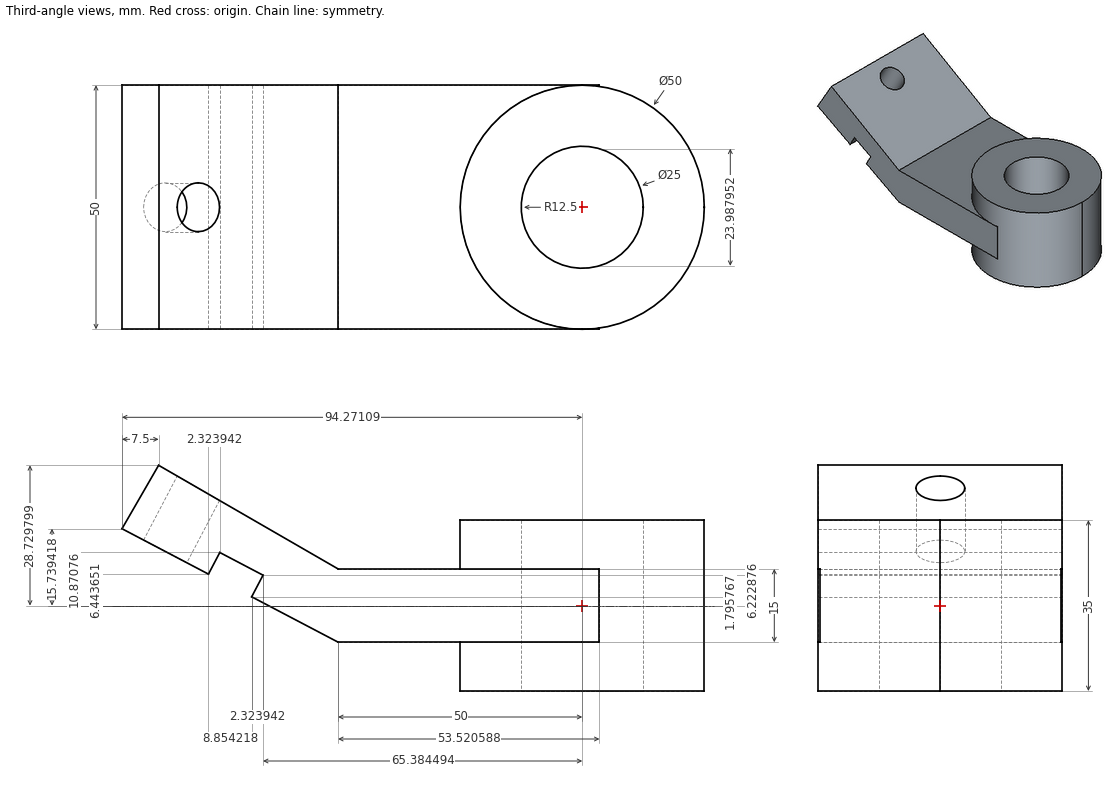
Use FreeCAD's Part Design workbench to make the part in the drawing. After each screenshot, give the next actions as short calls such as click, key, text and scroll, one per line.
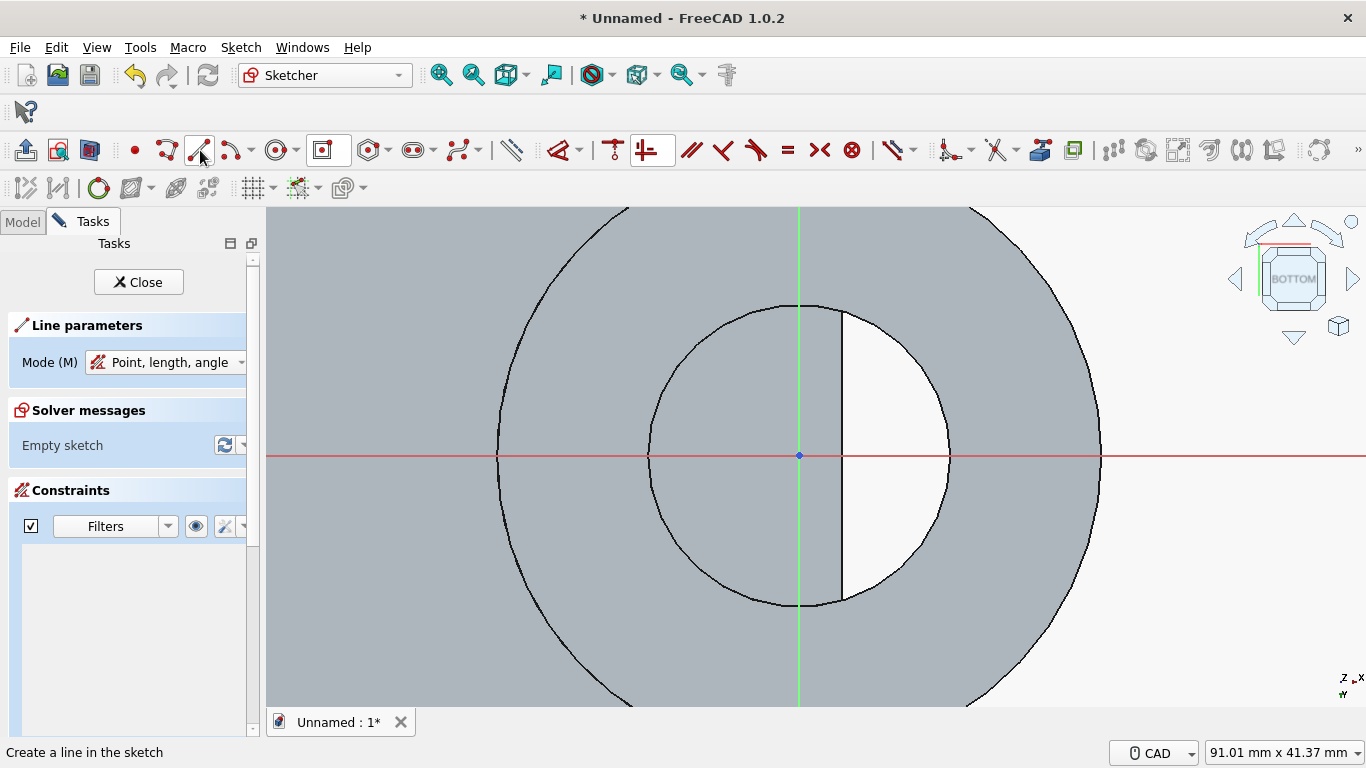
click(842, 601)
click(842, 311)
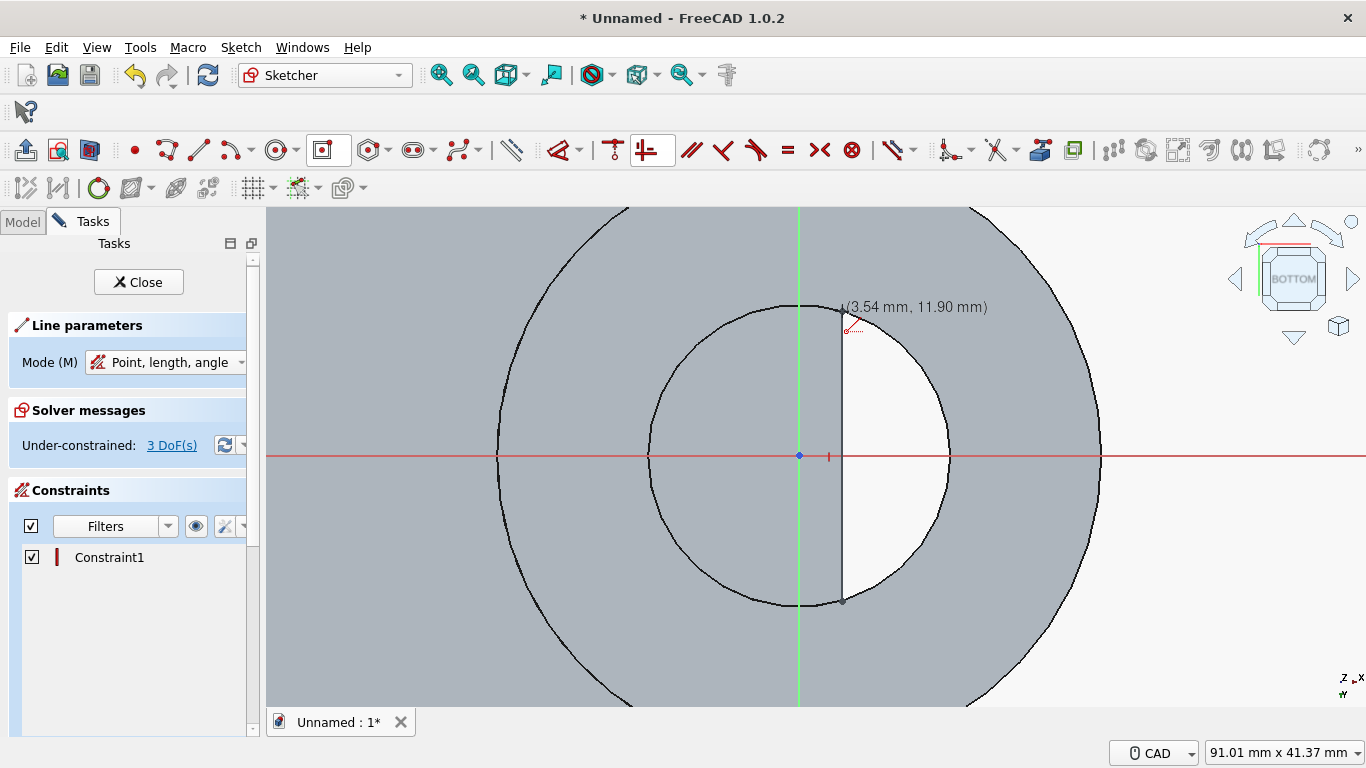
key(g)
key(3)
key(a)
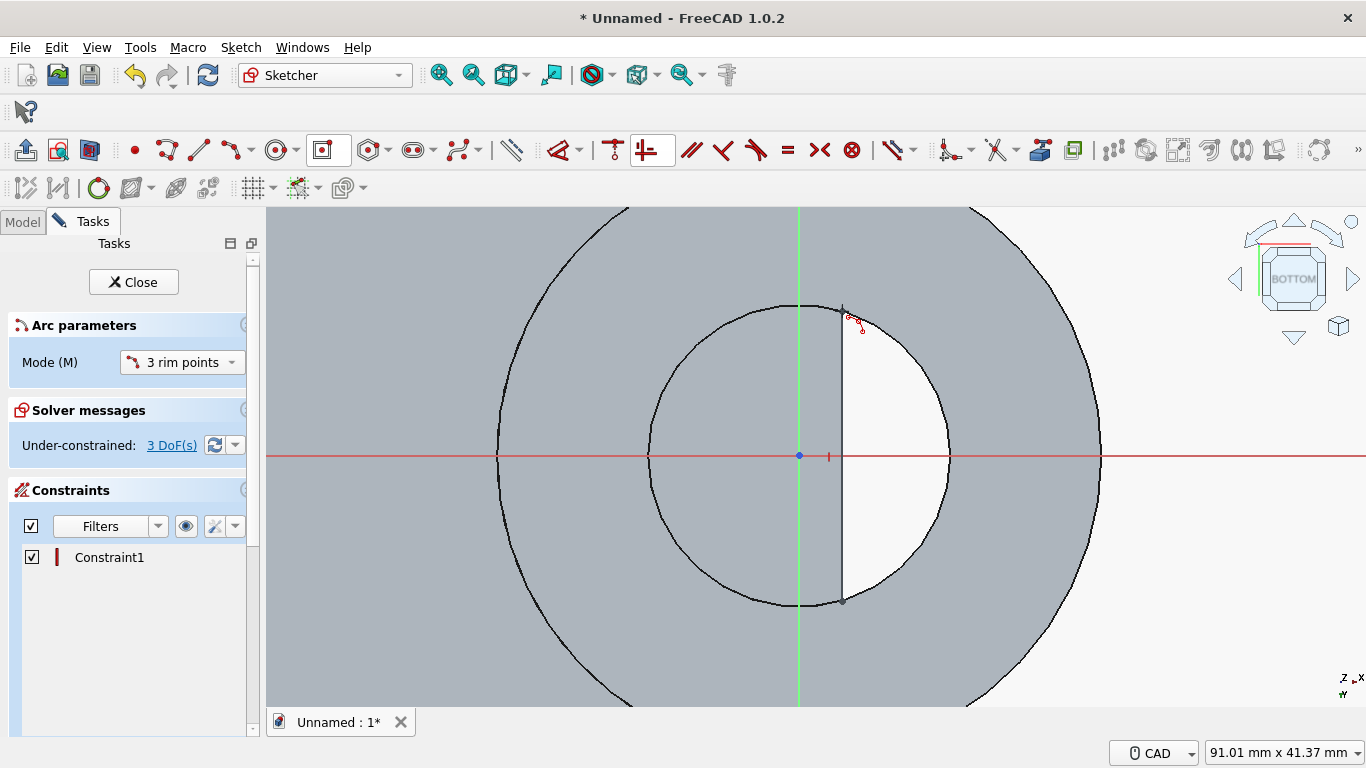
click(842, 312)
click(842, 602)
click(658, 401)
key(Escape)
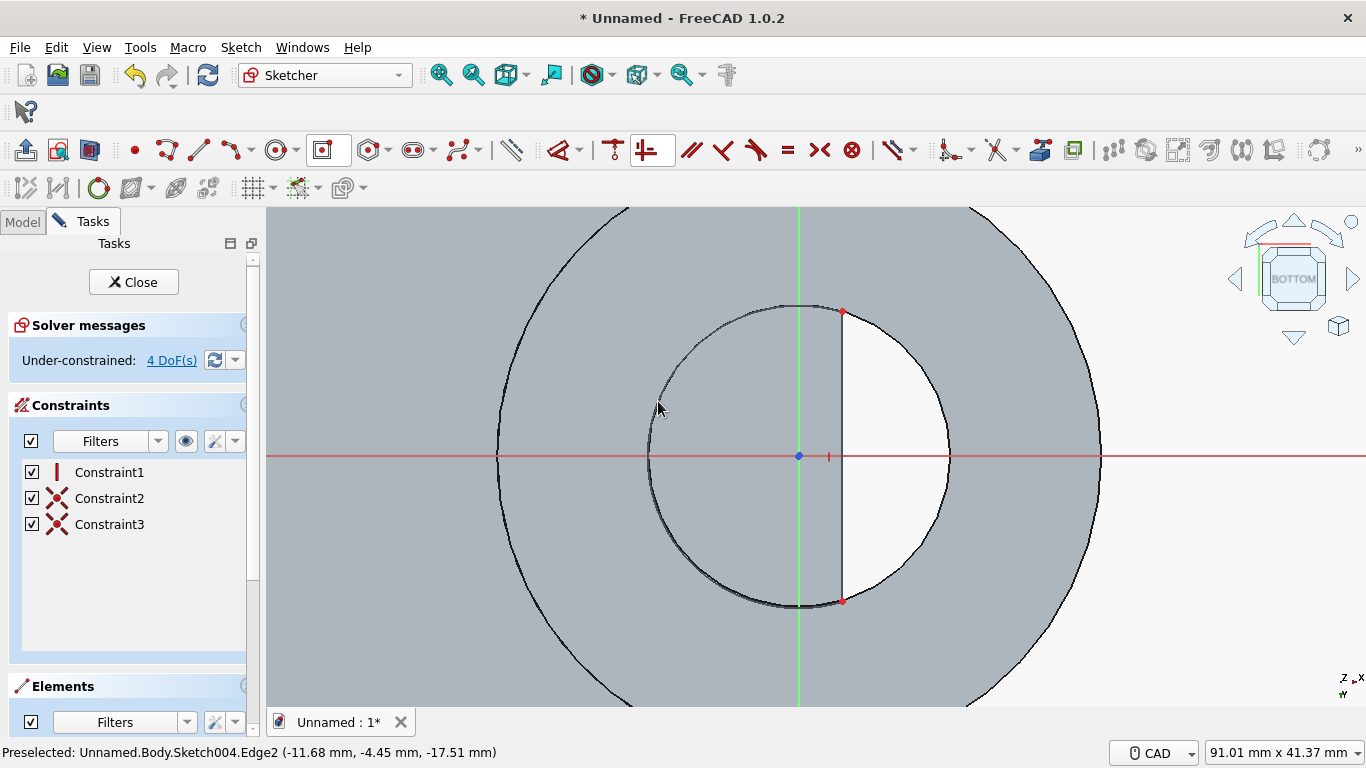
drag(789, 446, 809, 467)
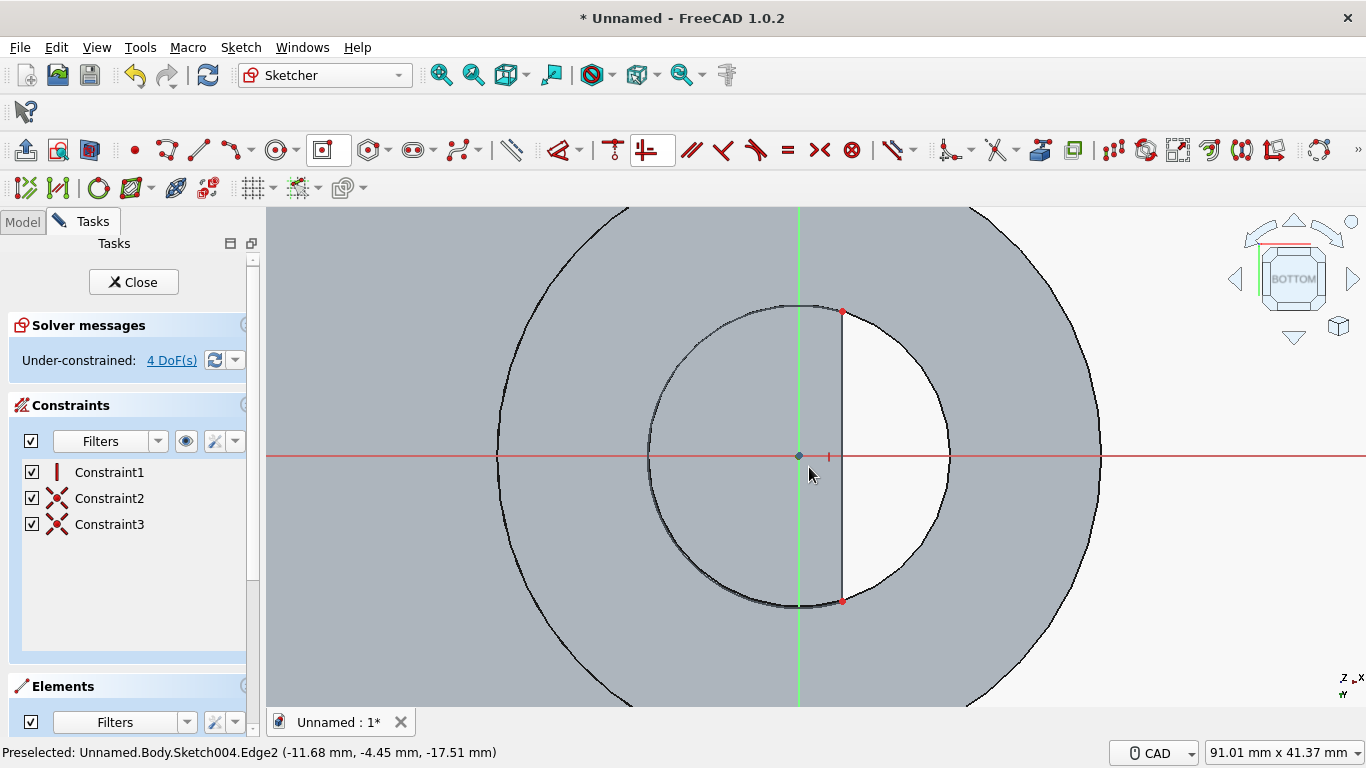
click(614, 150)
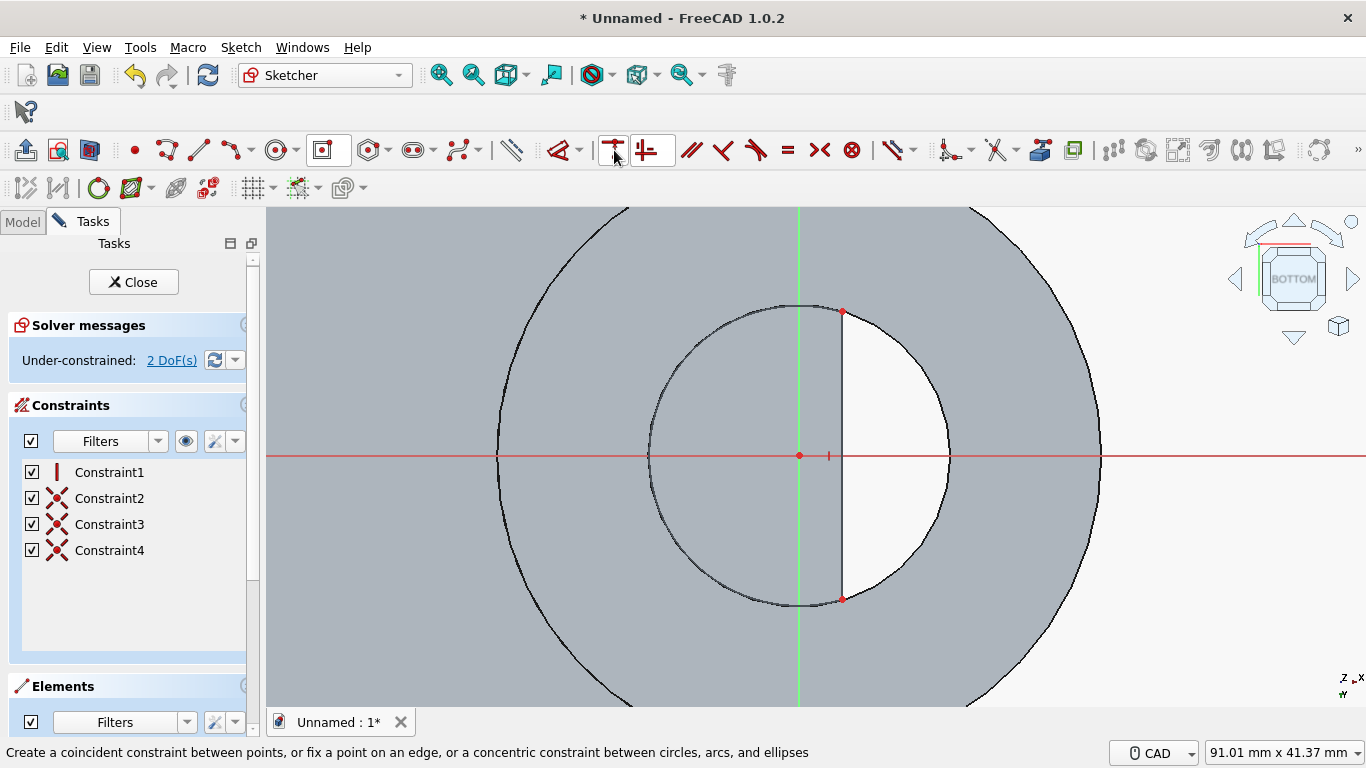
click(558, 150)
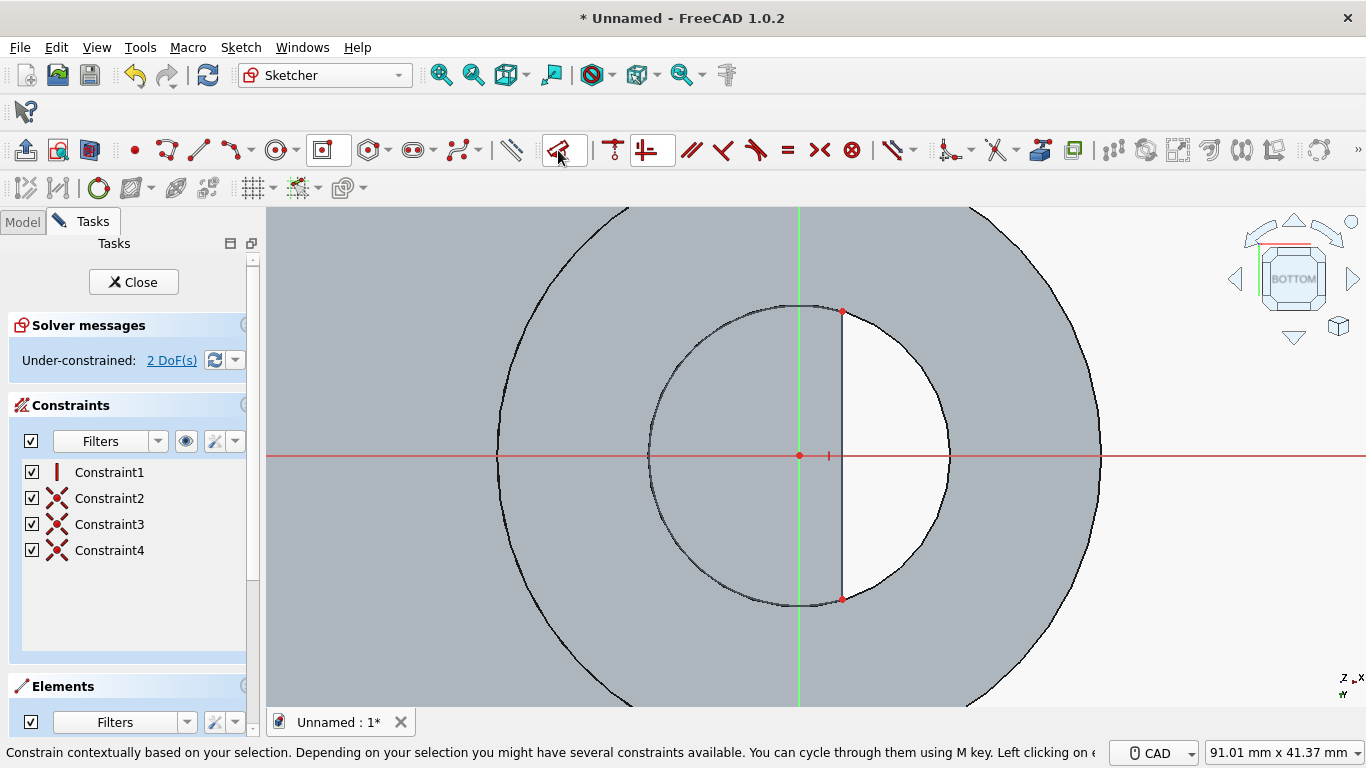
click(689, 354)
click(665, 332)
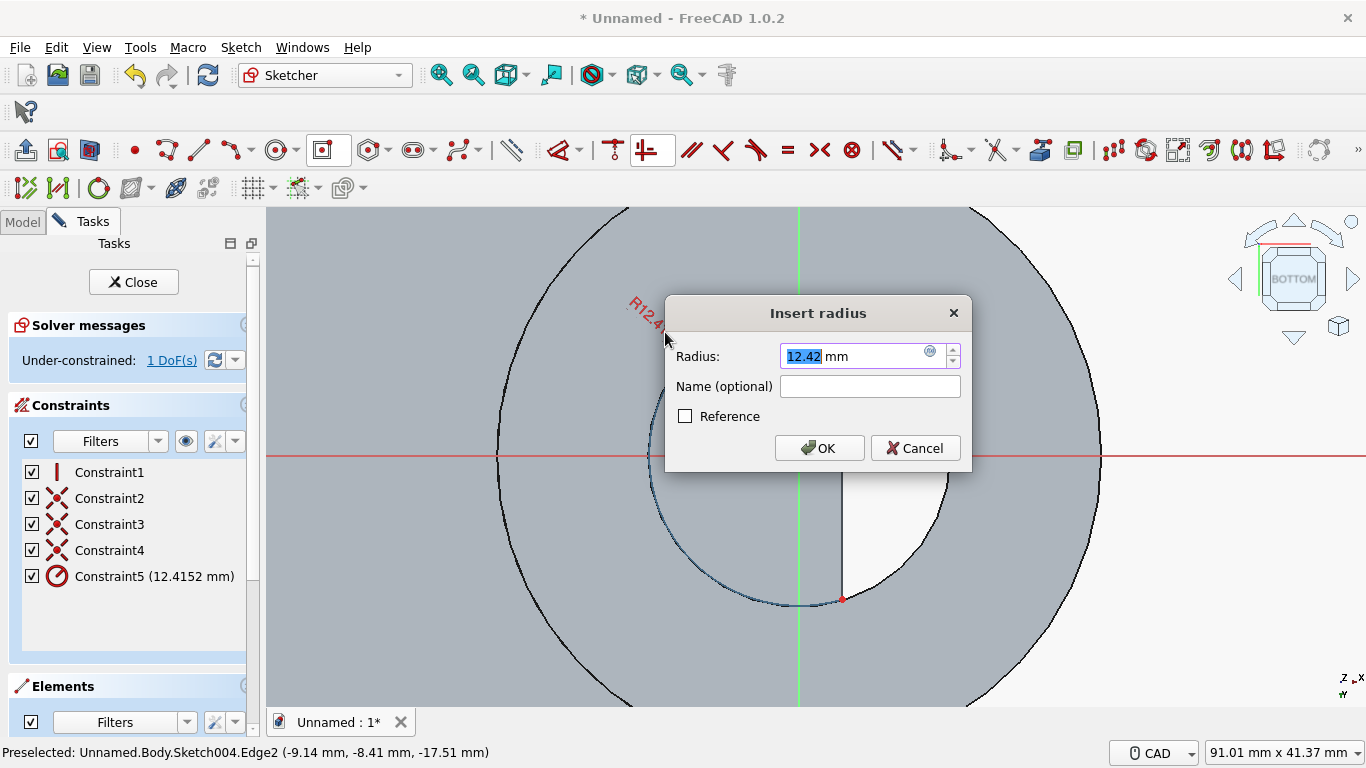
text(12.5)
key(Return)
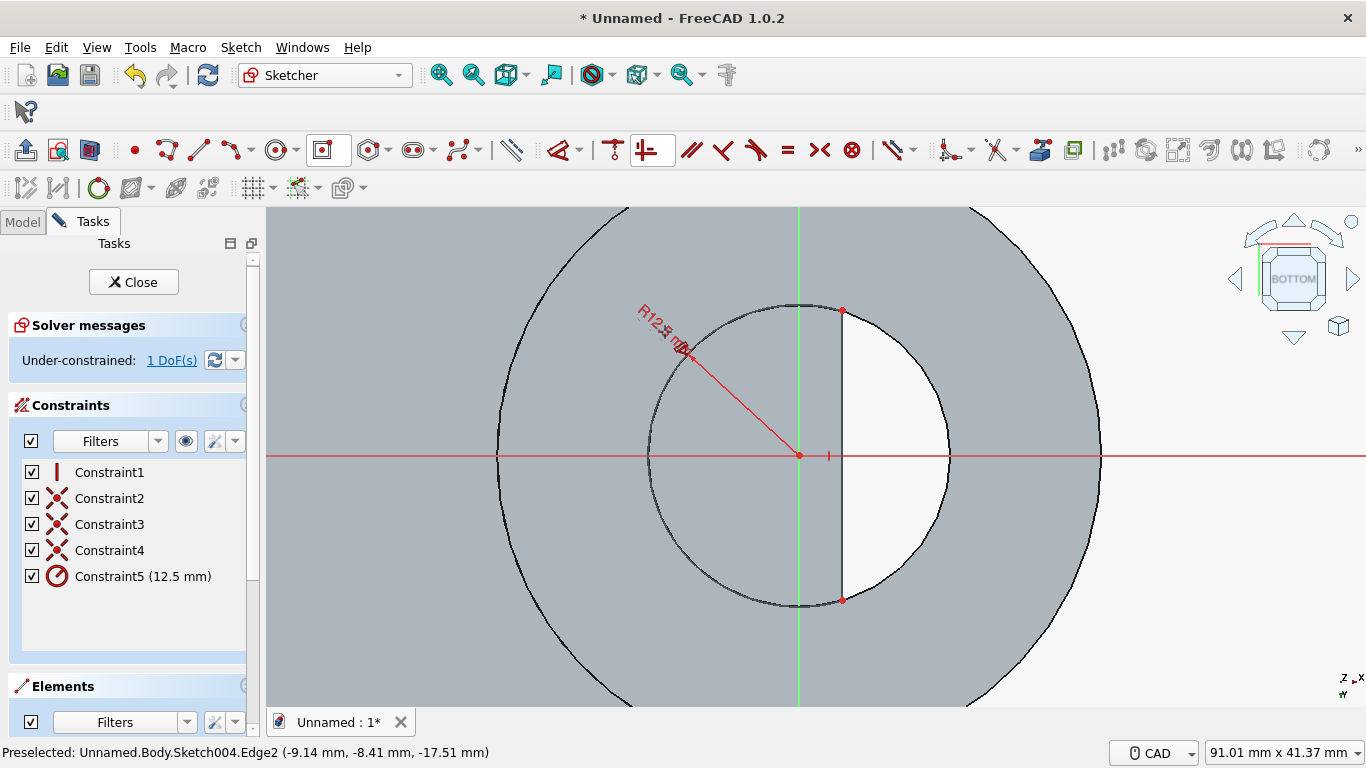
click(842, 514)
click(876, 389)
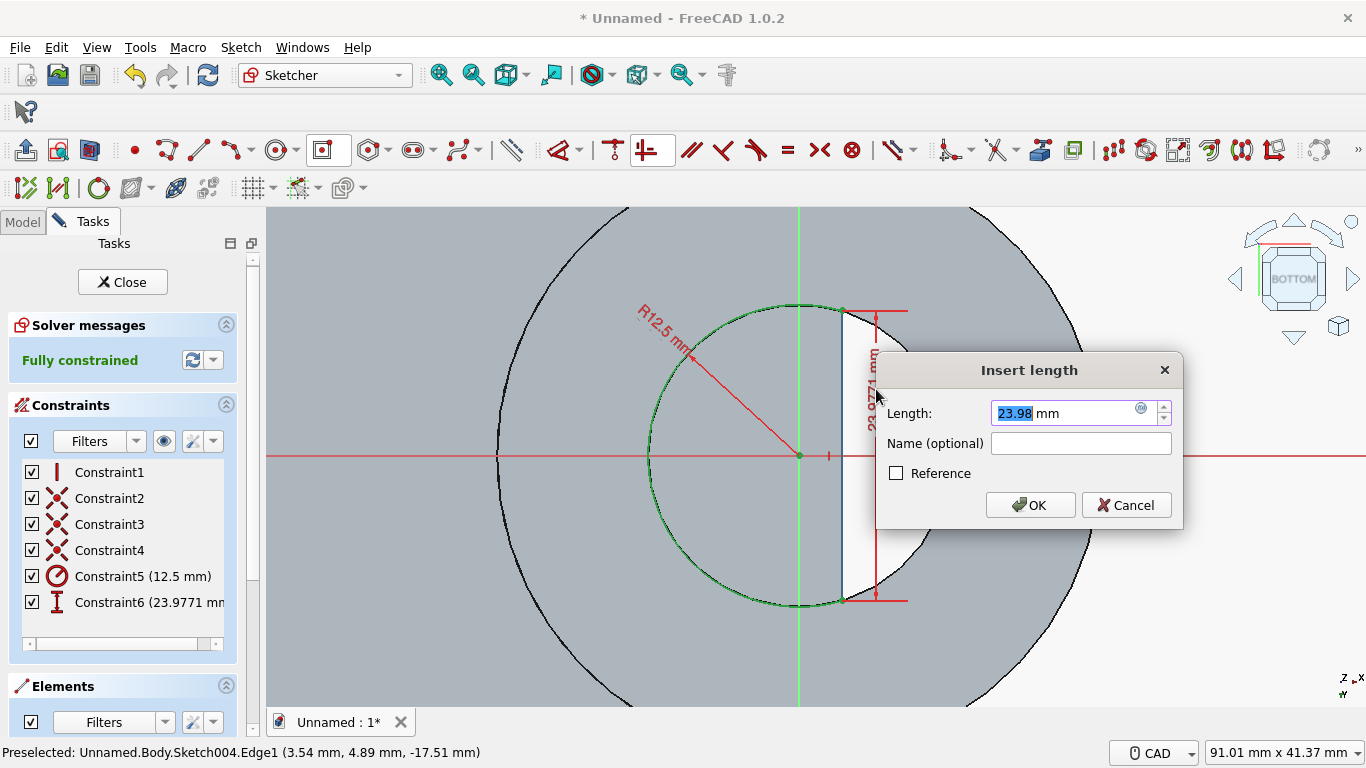
text(23.987952)
key(Return)
key(Escape)